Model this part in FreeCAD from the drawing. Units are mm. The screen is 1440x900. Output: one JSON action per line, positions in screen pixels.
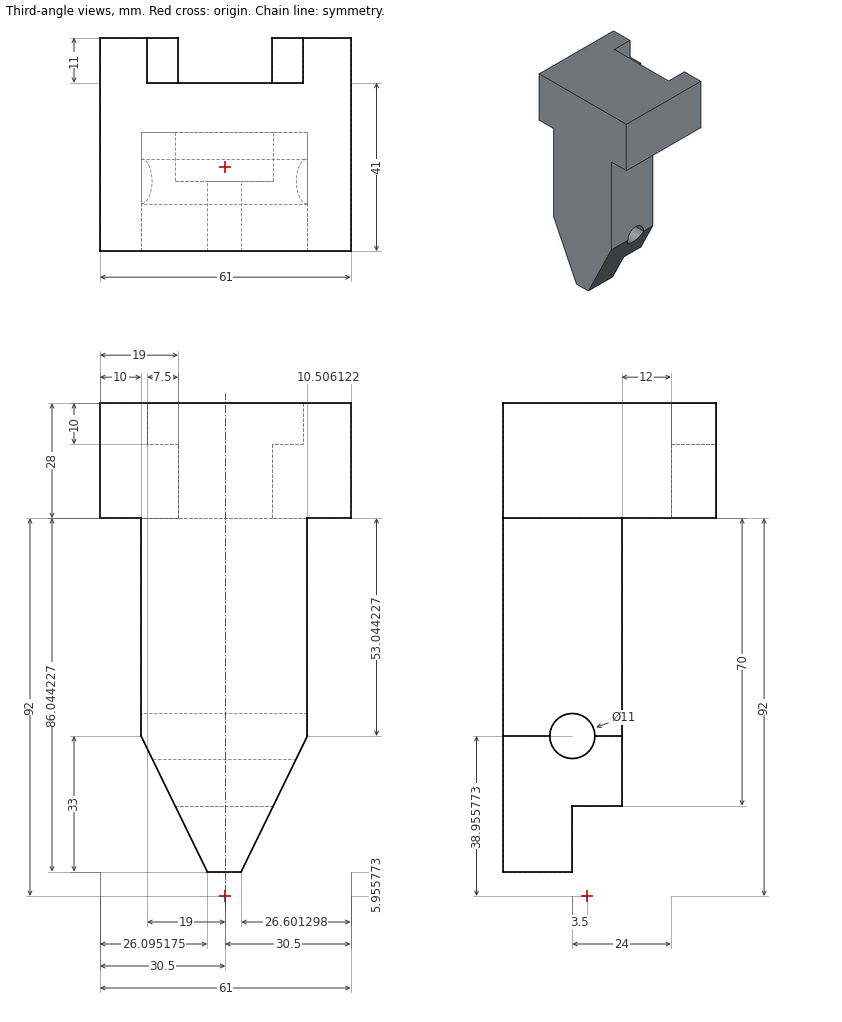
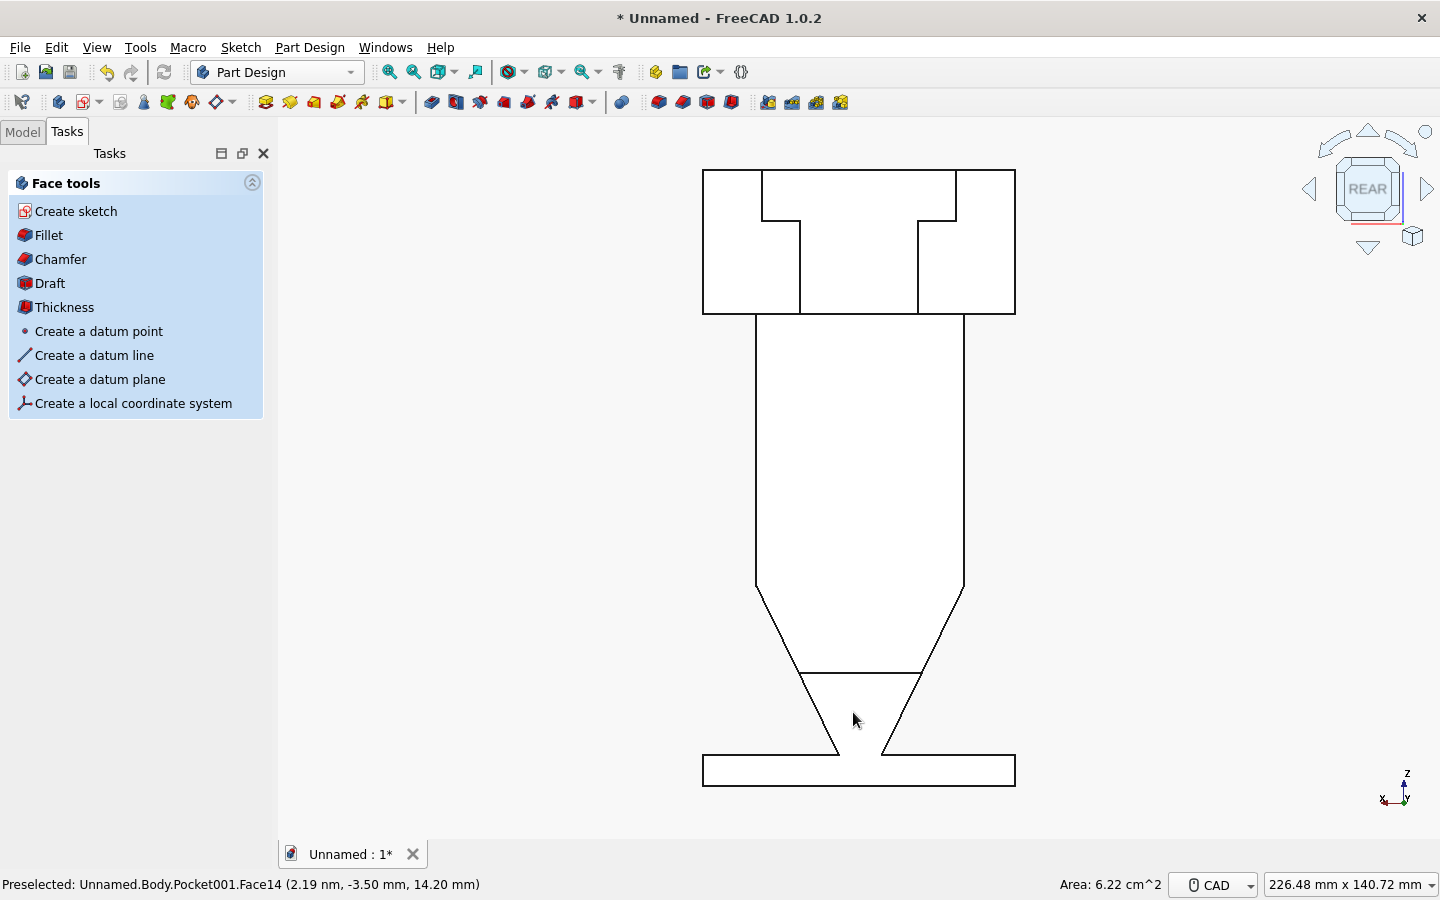
{"action": "left_click", "coordinate": [84, 102]}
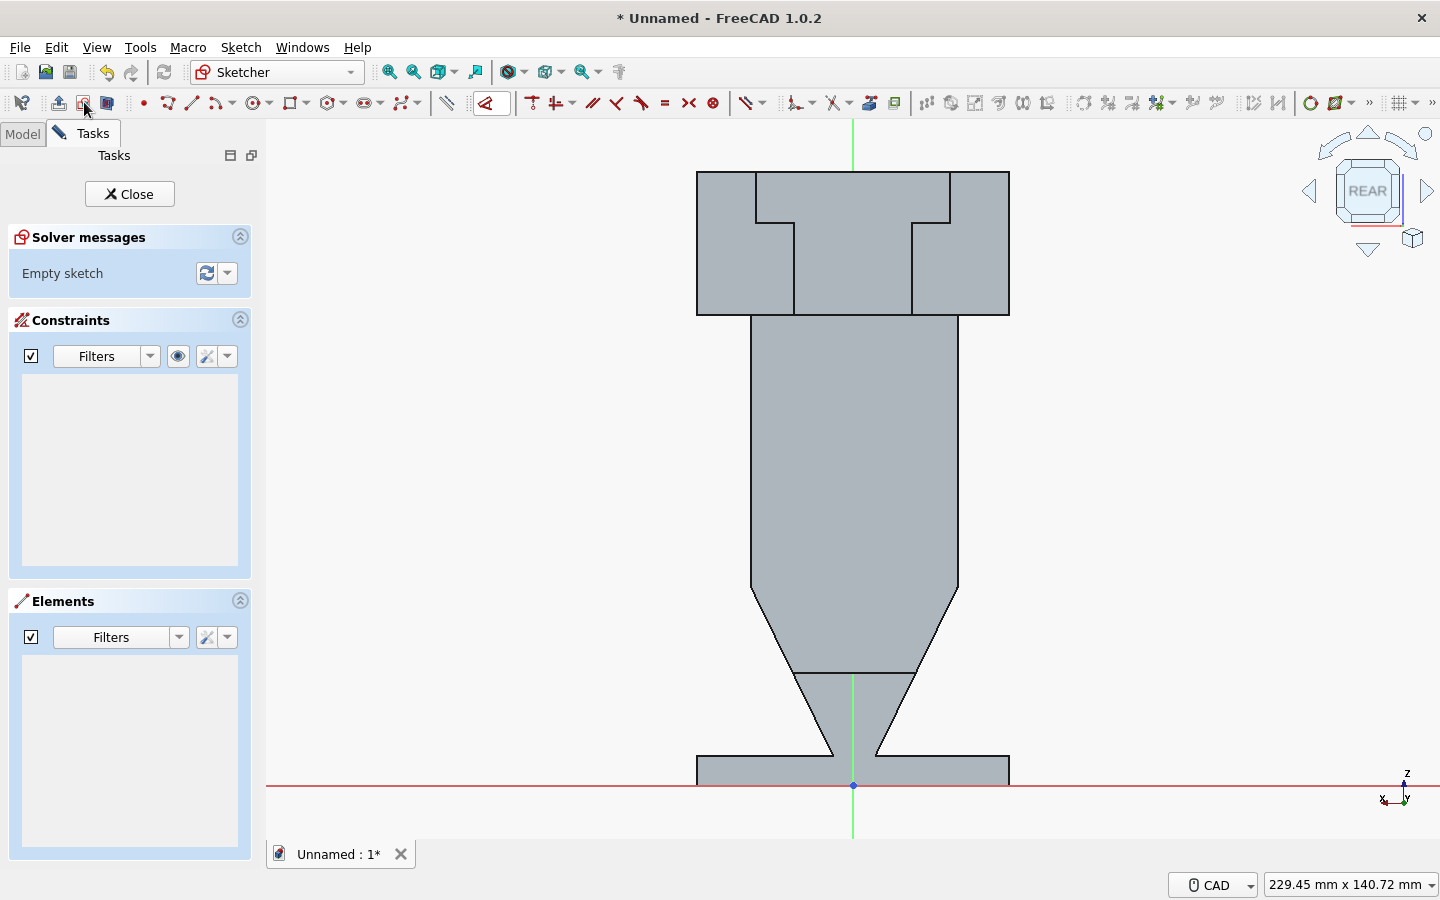
{"action": "scroll", "coordinate": [909, 811], "scroll_direction": "up", "scroll_amount": 4}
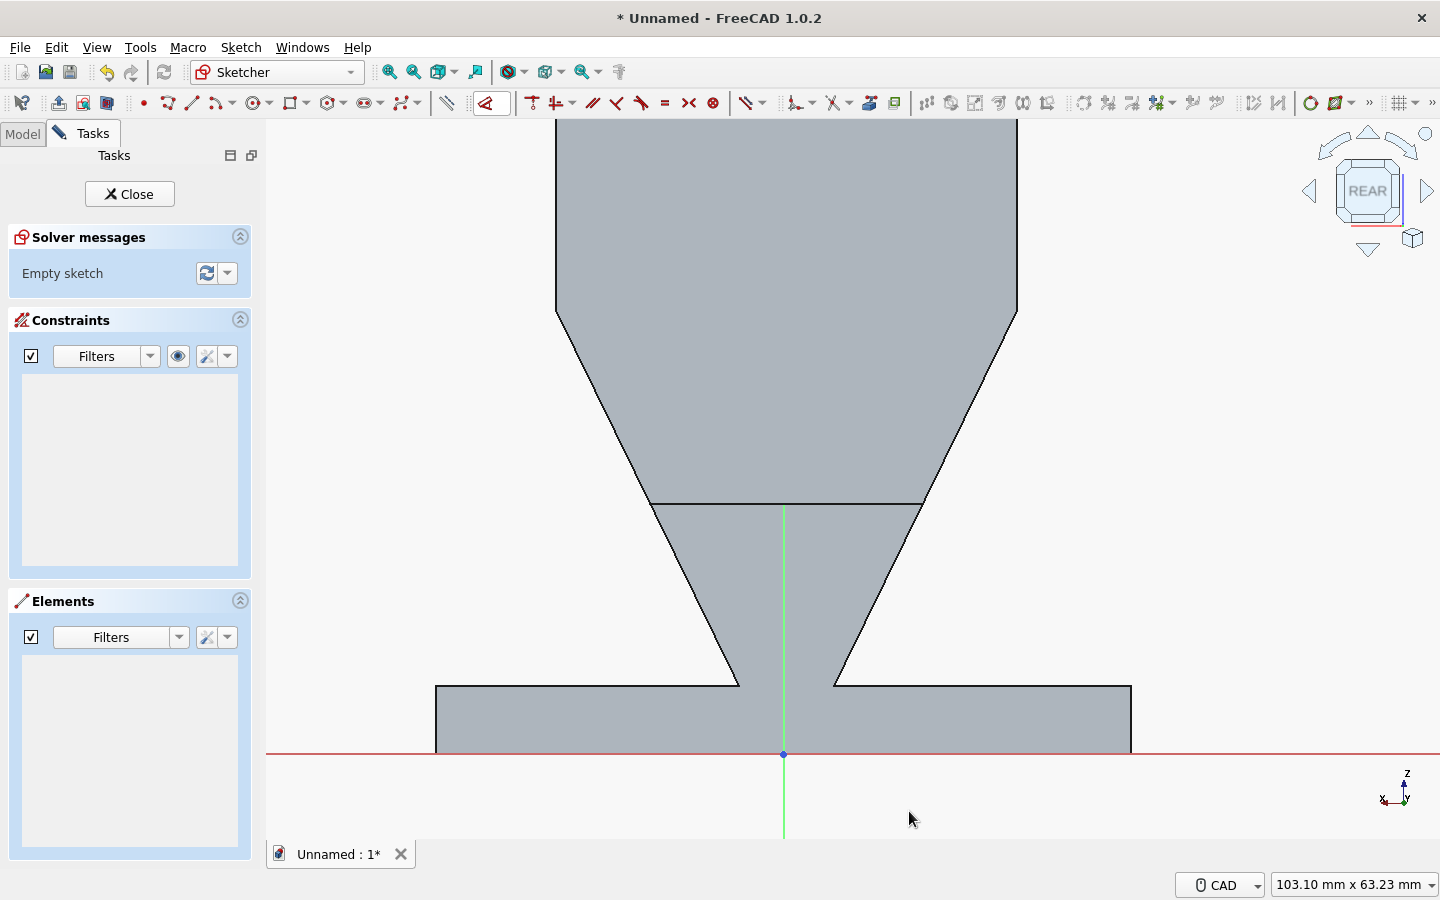
{"action": "left_click", "coordinate": [290, 104]}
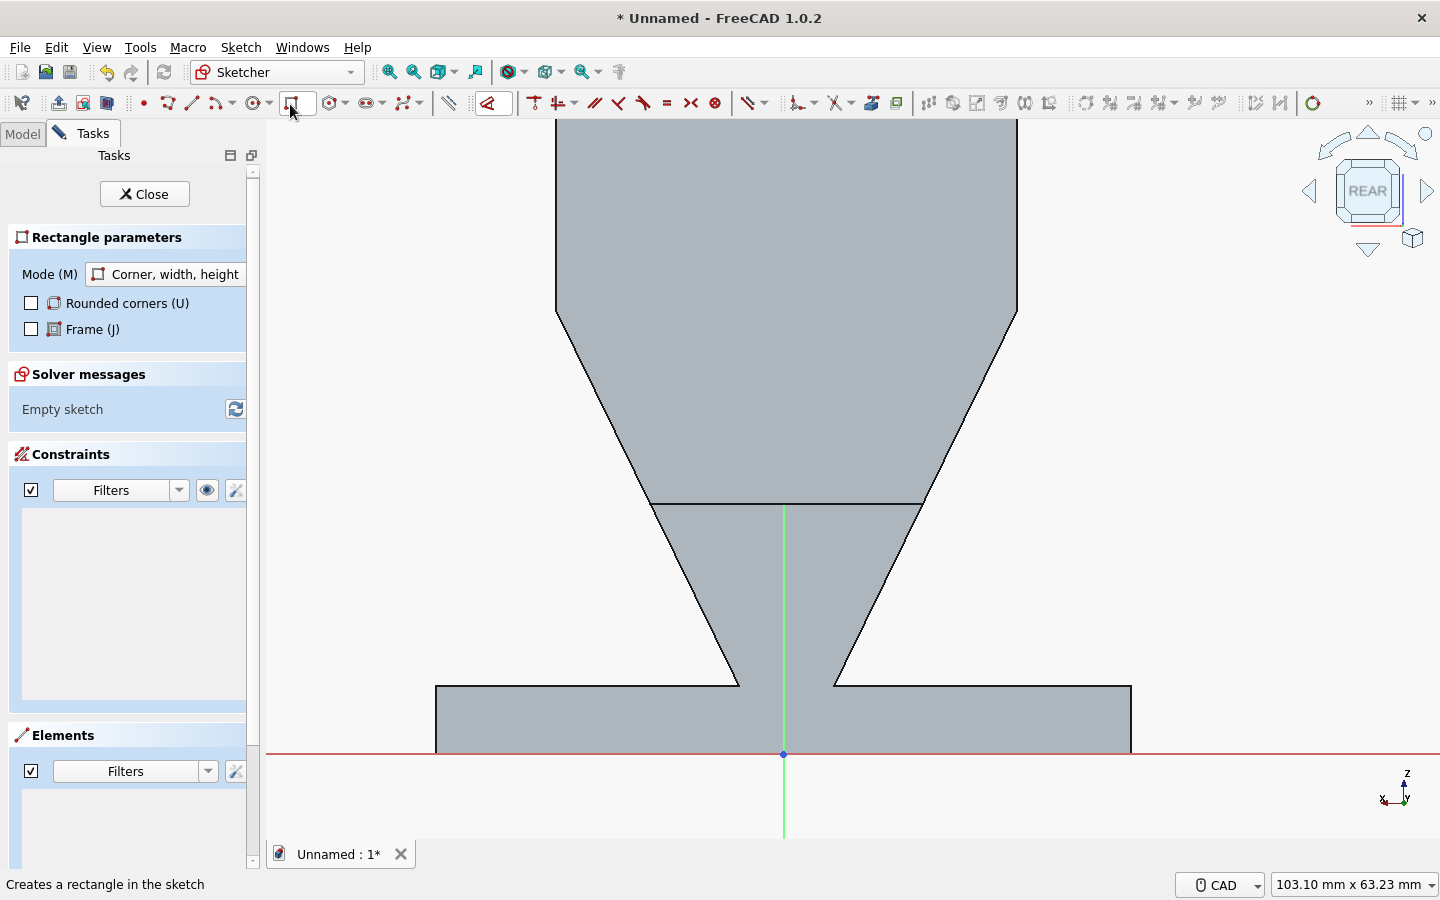
{"action": "left_click", "coordinate": [436, 686]}
{"action": "left_click", "coordinate": [1131, 754]}
{"action": "key", "text": "Escape"}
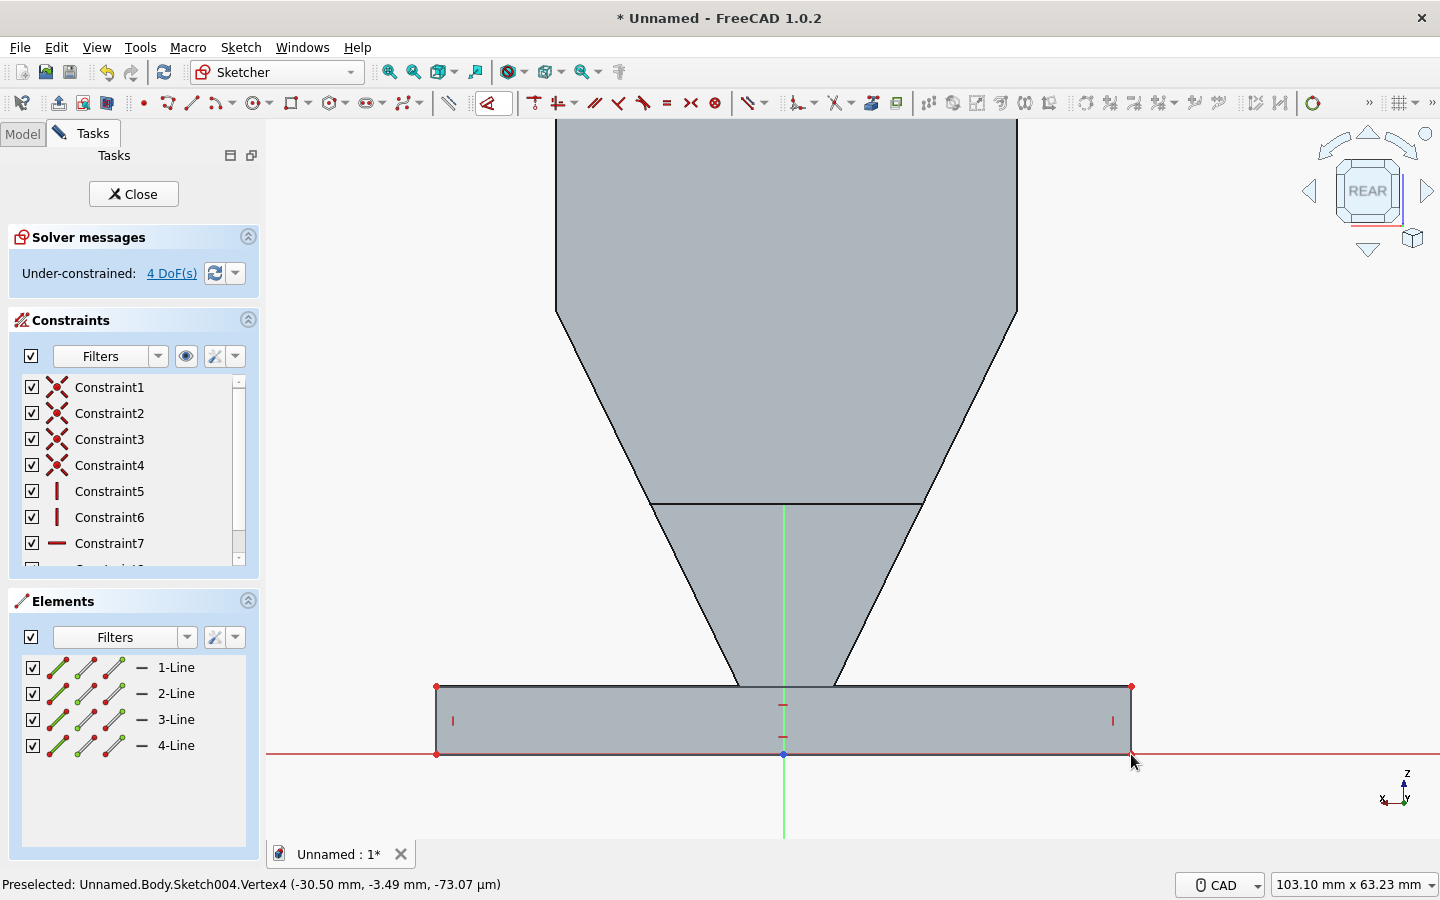
{"action": "left_click", "coordinate": [436, 755]}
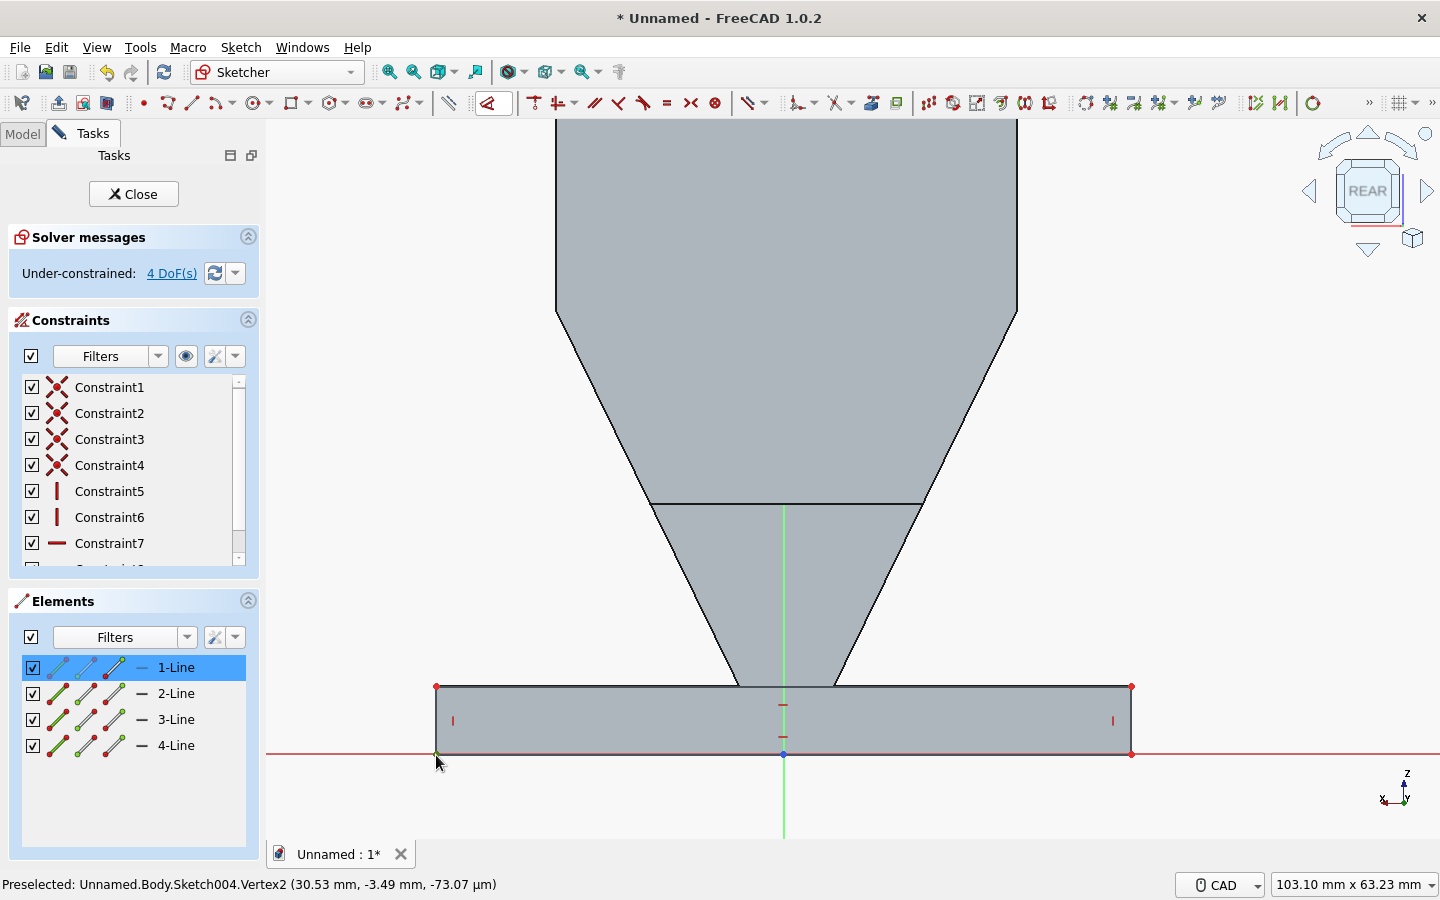
{"action": "left_click", "coordinate": [364, 754]}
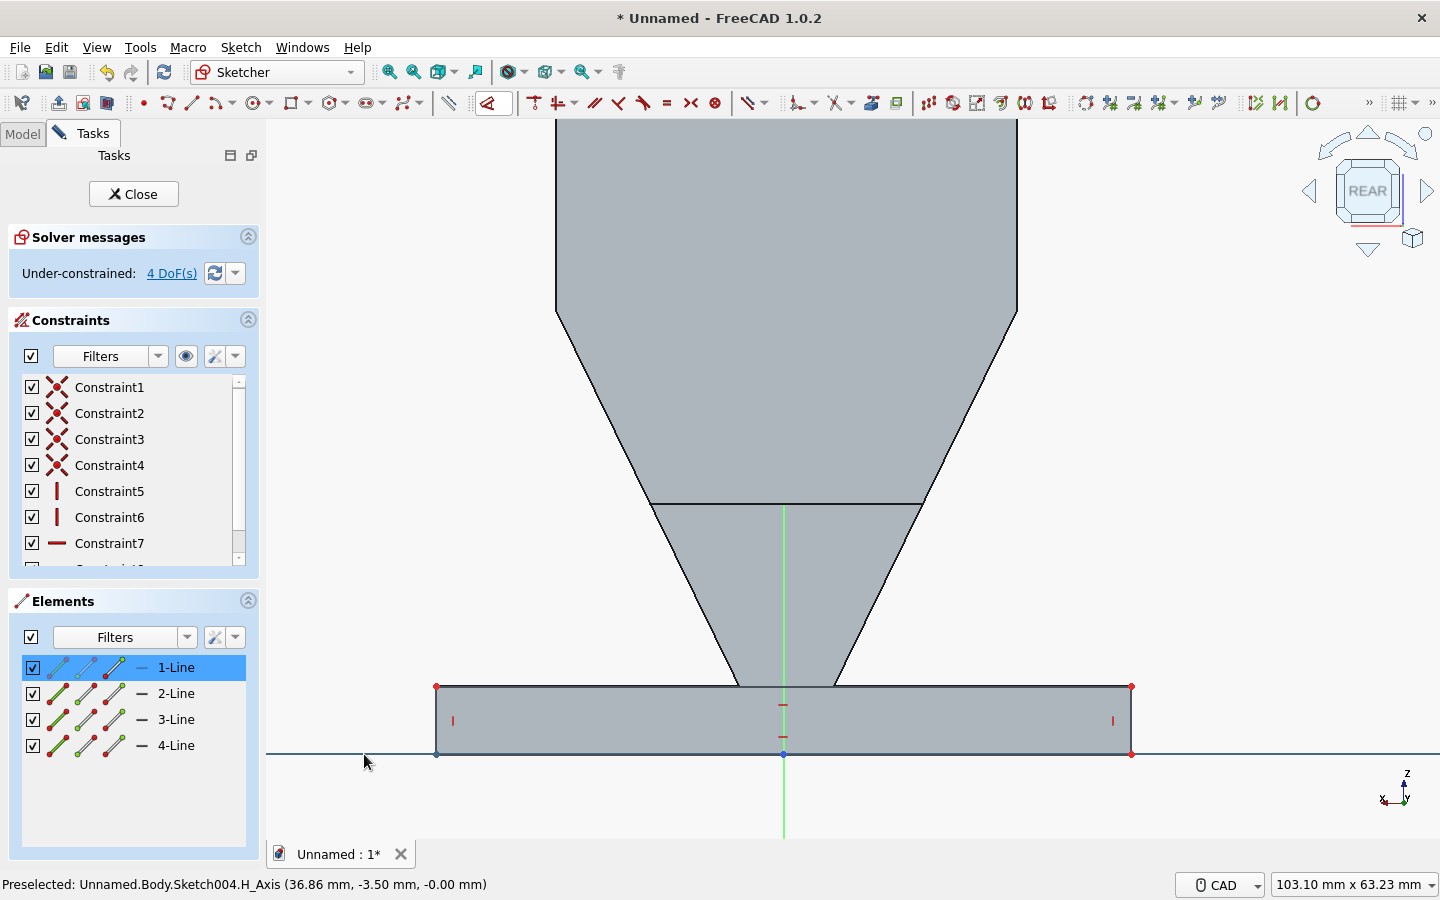
{"action": "left_click", "coordinate": [534, 104]}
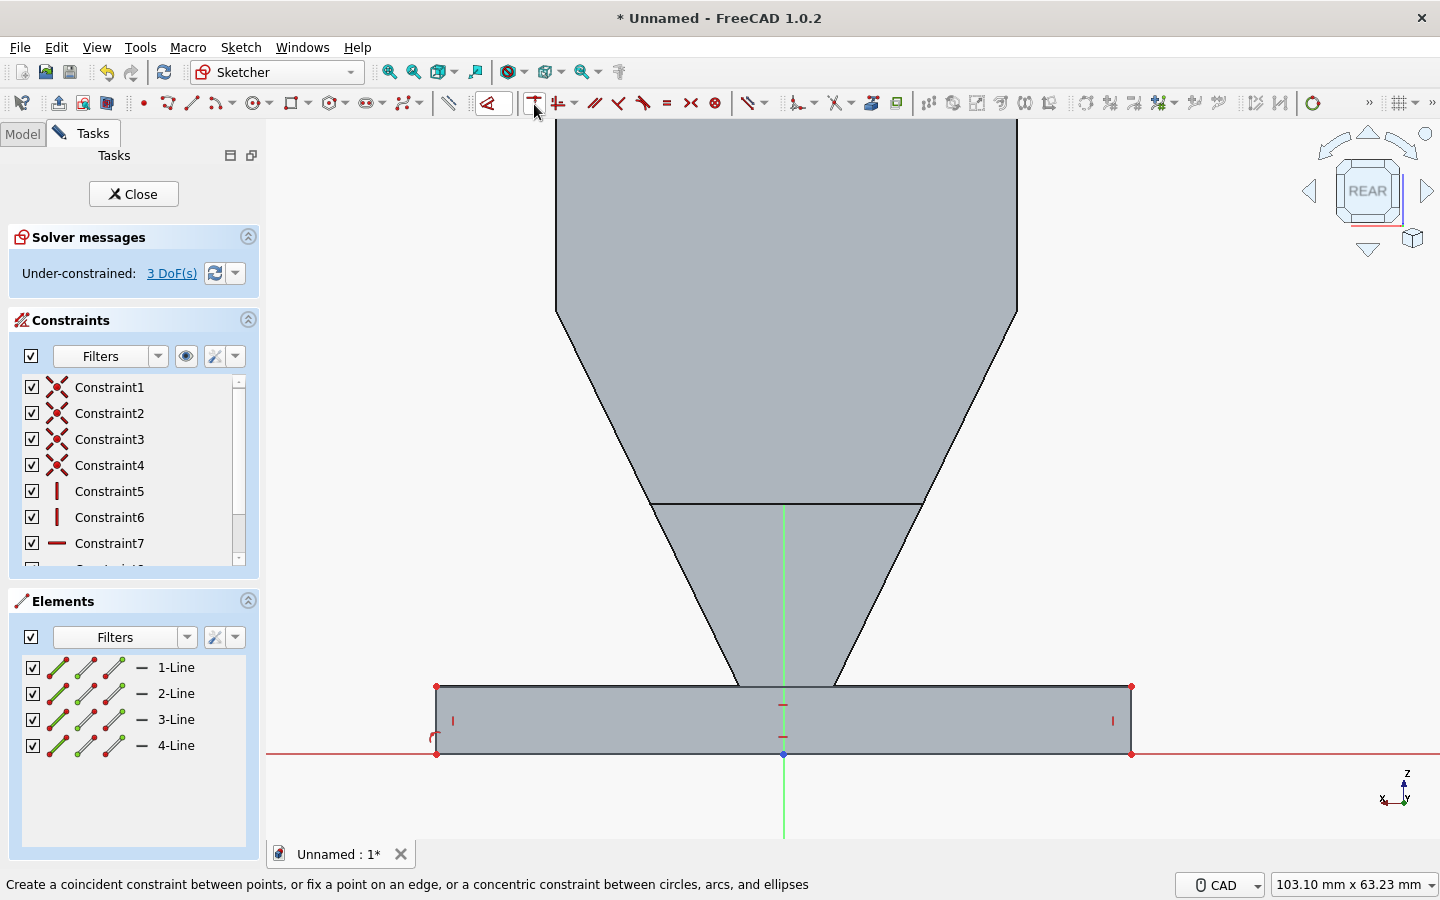
{"action": "left_click", "coordinate": [645, 754]}